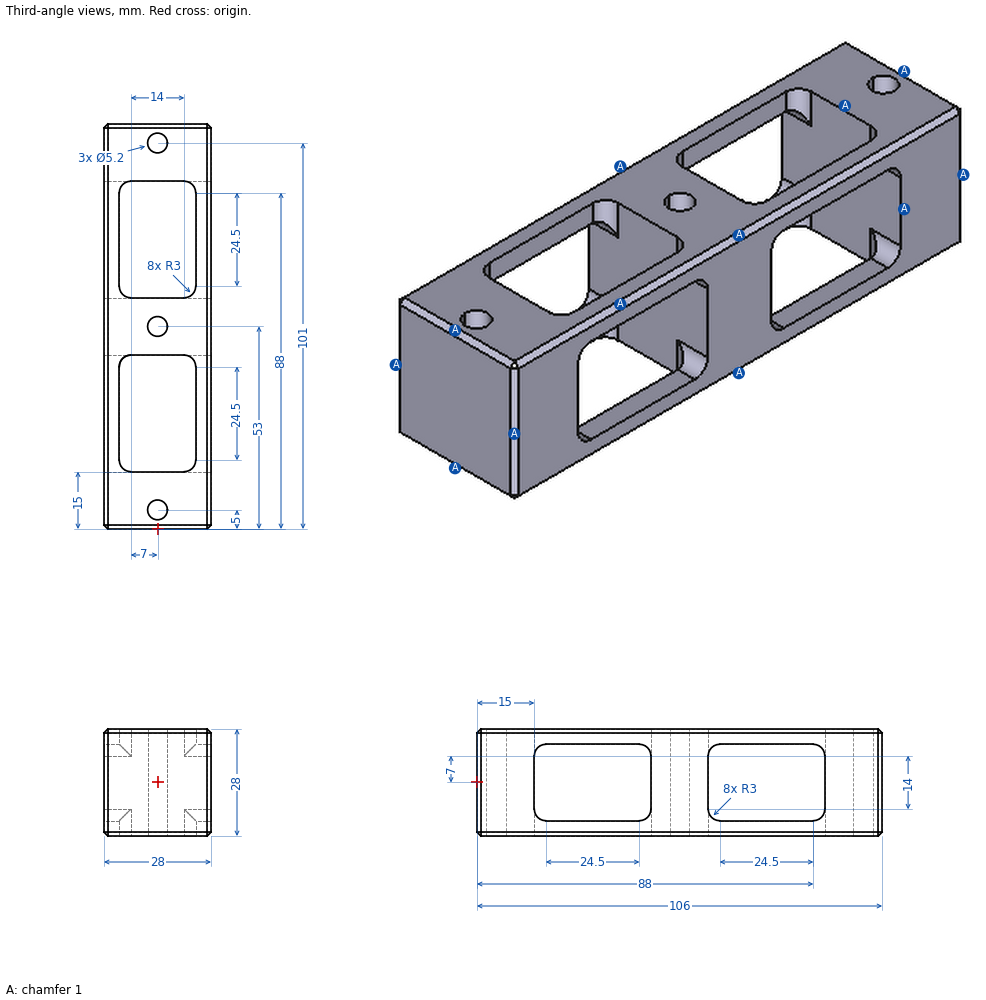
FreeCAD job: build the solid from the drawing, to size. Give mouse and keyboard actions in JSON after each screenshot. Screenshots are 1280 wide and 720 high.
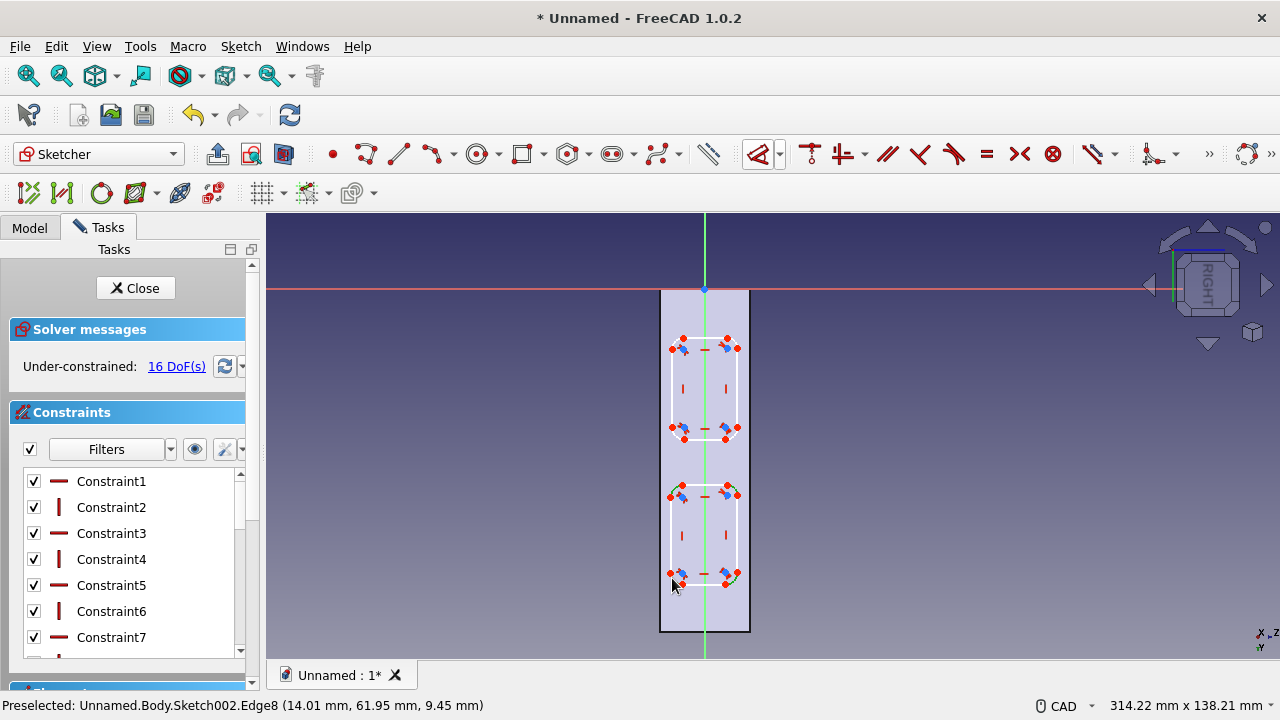
{"action": "scroll", "coordinate": [678, 339], "scroll_direction": "up", "scroll_amount": 5}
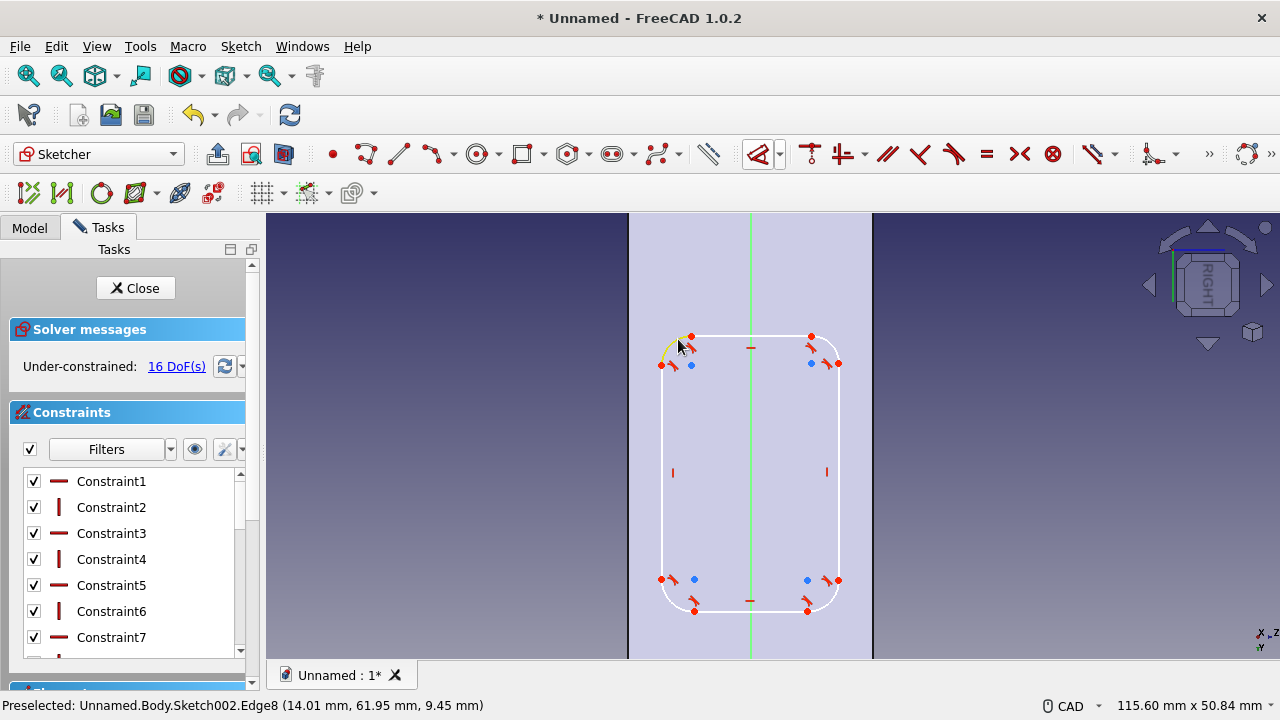
{"action": "left_click", "coordinate": [678, 339]}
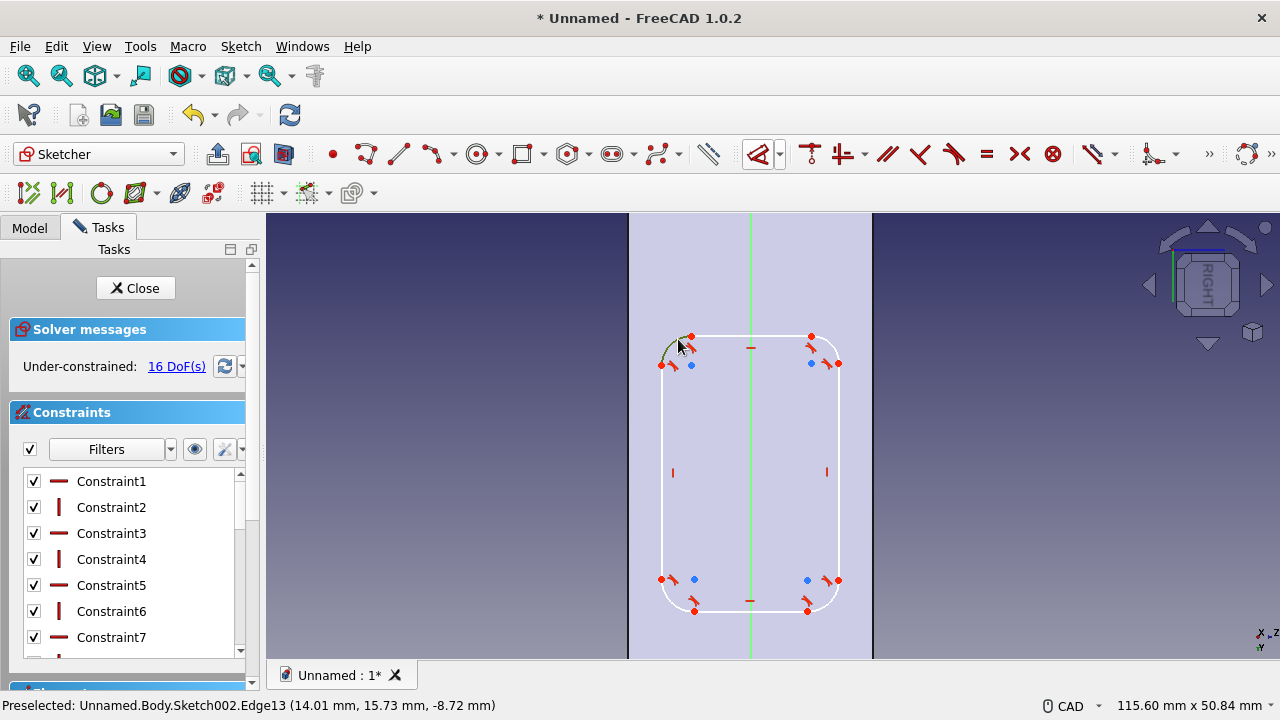
{"action": "left_click", "coordinate": [665, 594]}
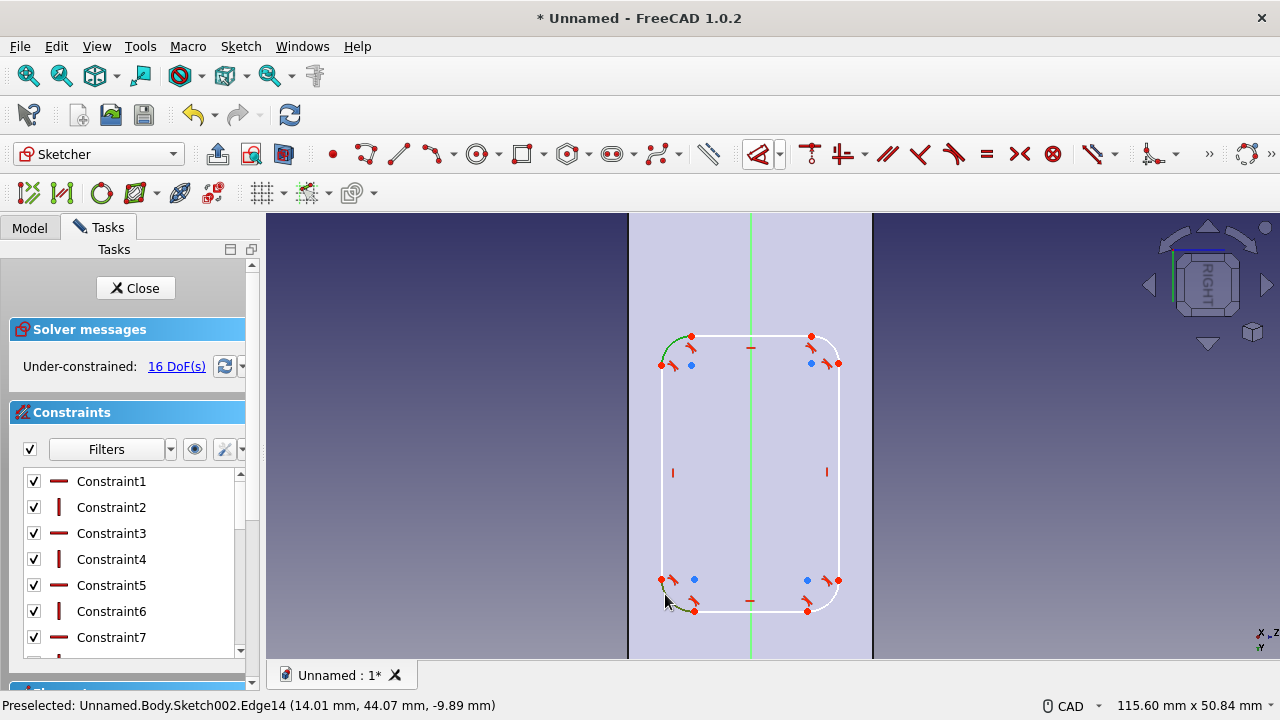
{"action": "left_click", "coordinate": [822, 608]}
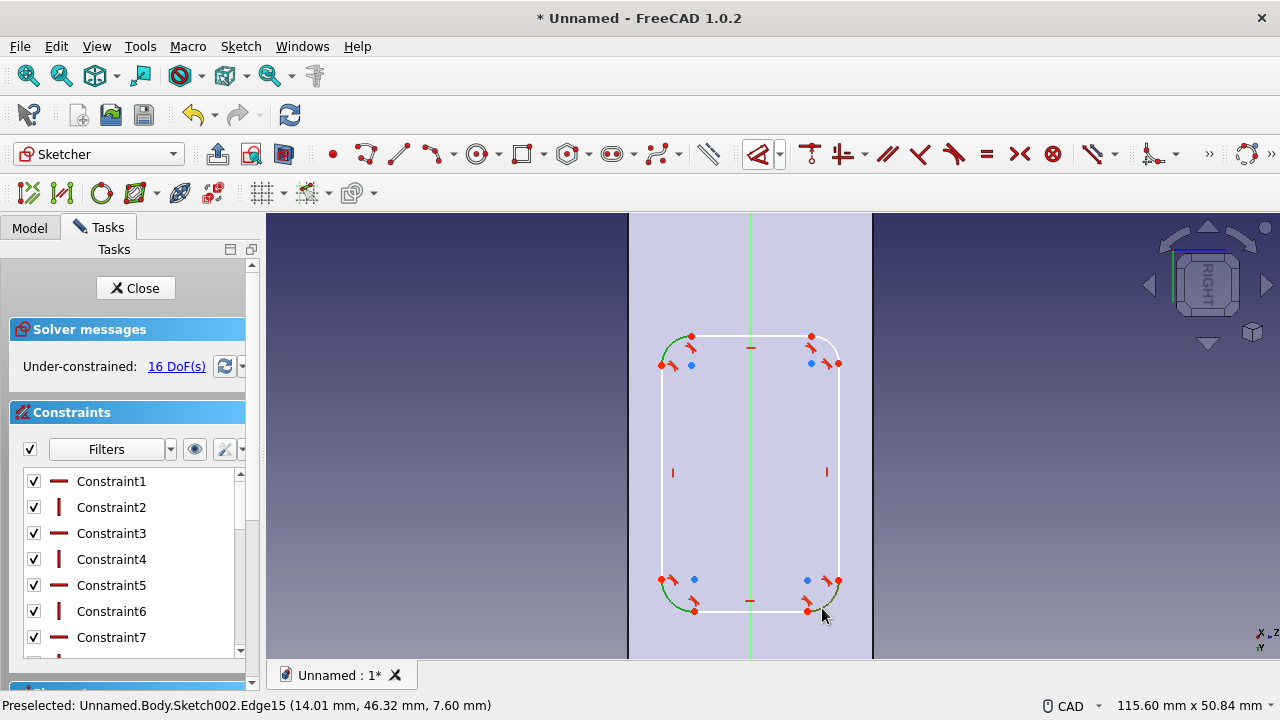
{"action": "left_click", "coordinate": [836, 351]}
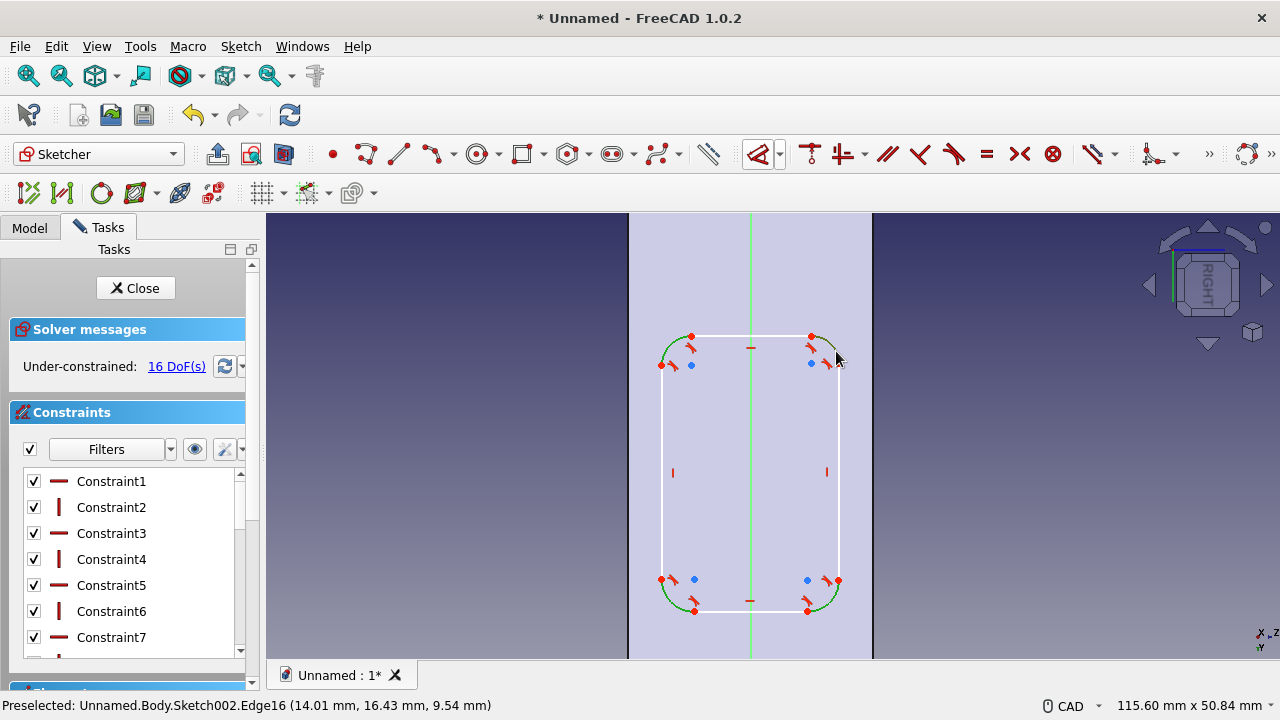
{"action": "left_click", "coordinate": [987, 154]}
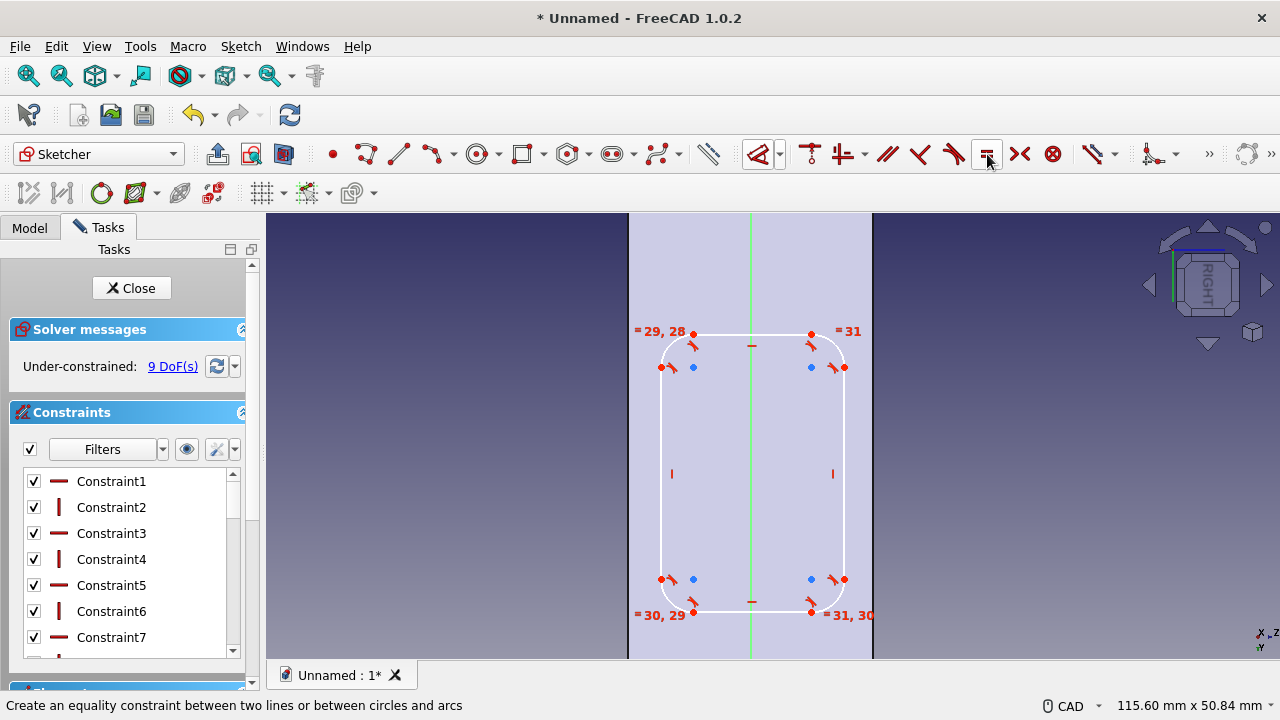
{"action": "scroll", "coordinate": [678, 339], "scroll_direction": "down", "scroll_amount": 5}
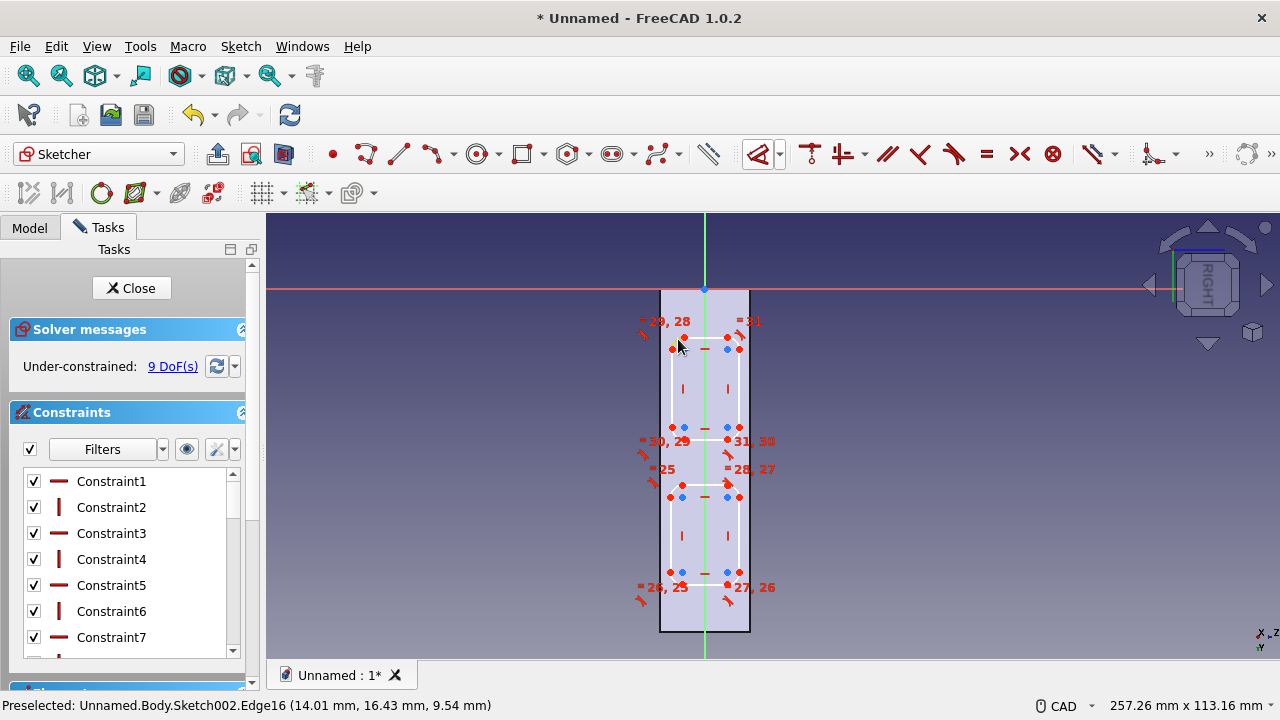
{"action": "scroll", "coordinate": [677, 486], "scroll_direction": "up", "scroll_amount": 8}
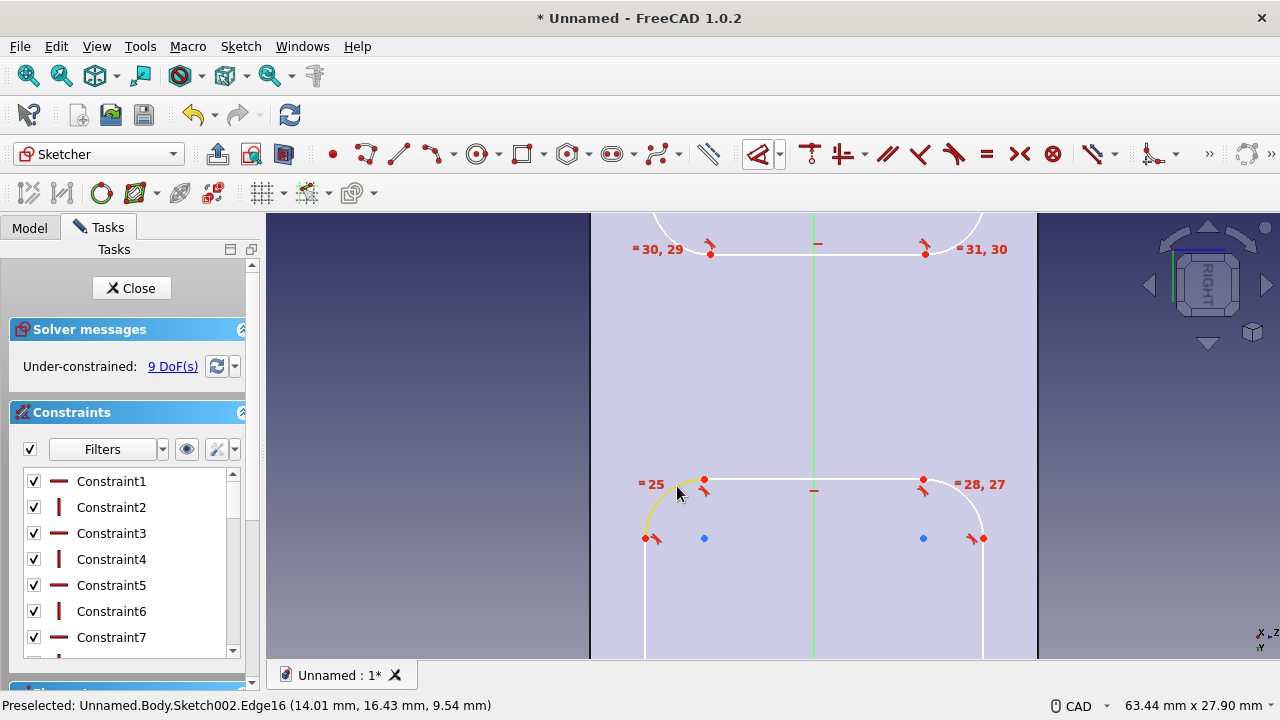
{"action": "left_click", "coordinate": [678, 486]}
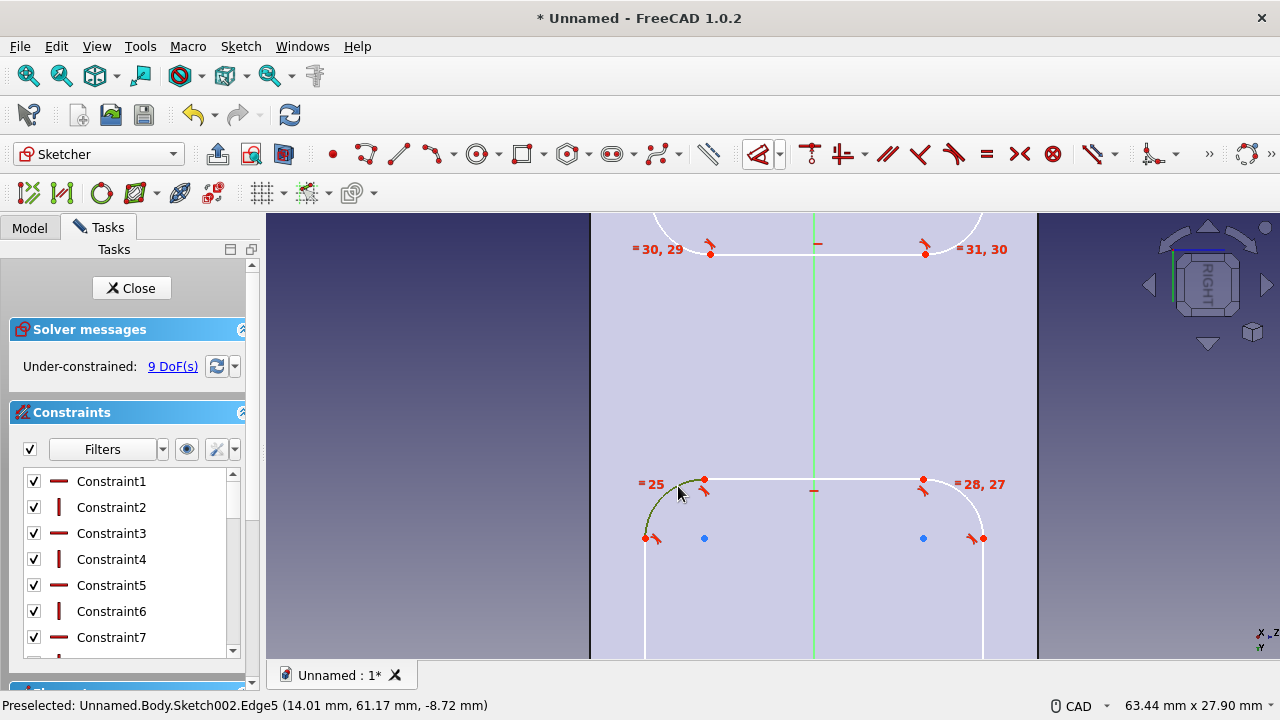
{"action": "left_click", "coordinate": [780, 154]}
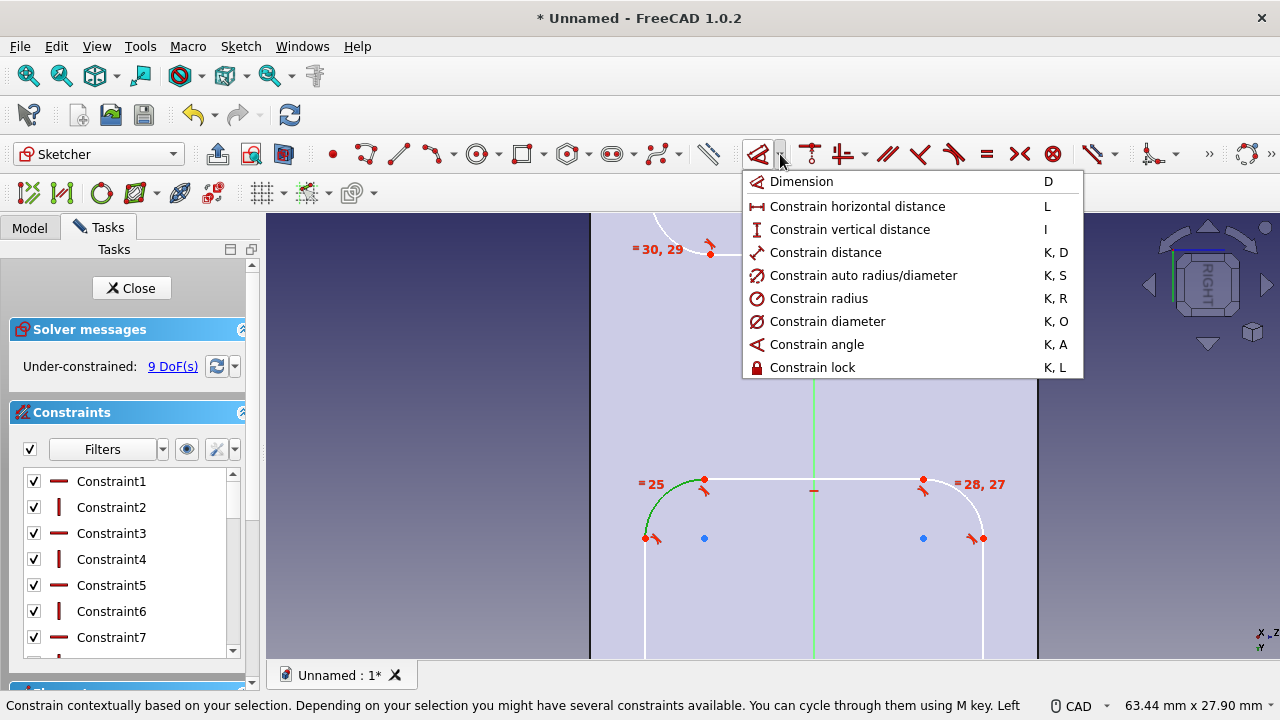
{"action": "left_click", "coordinate": [913, 298]}